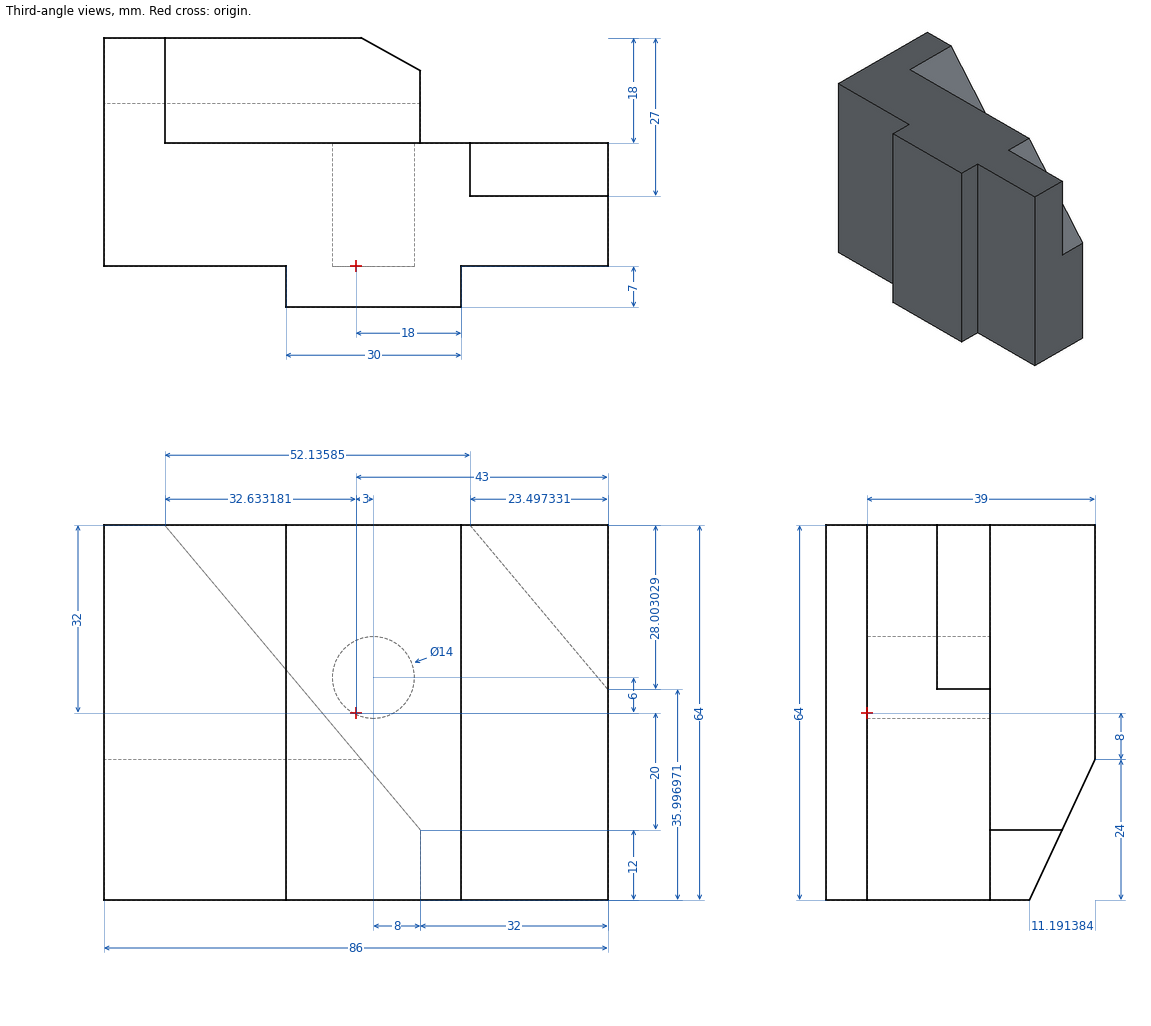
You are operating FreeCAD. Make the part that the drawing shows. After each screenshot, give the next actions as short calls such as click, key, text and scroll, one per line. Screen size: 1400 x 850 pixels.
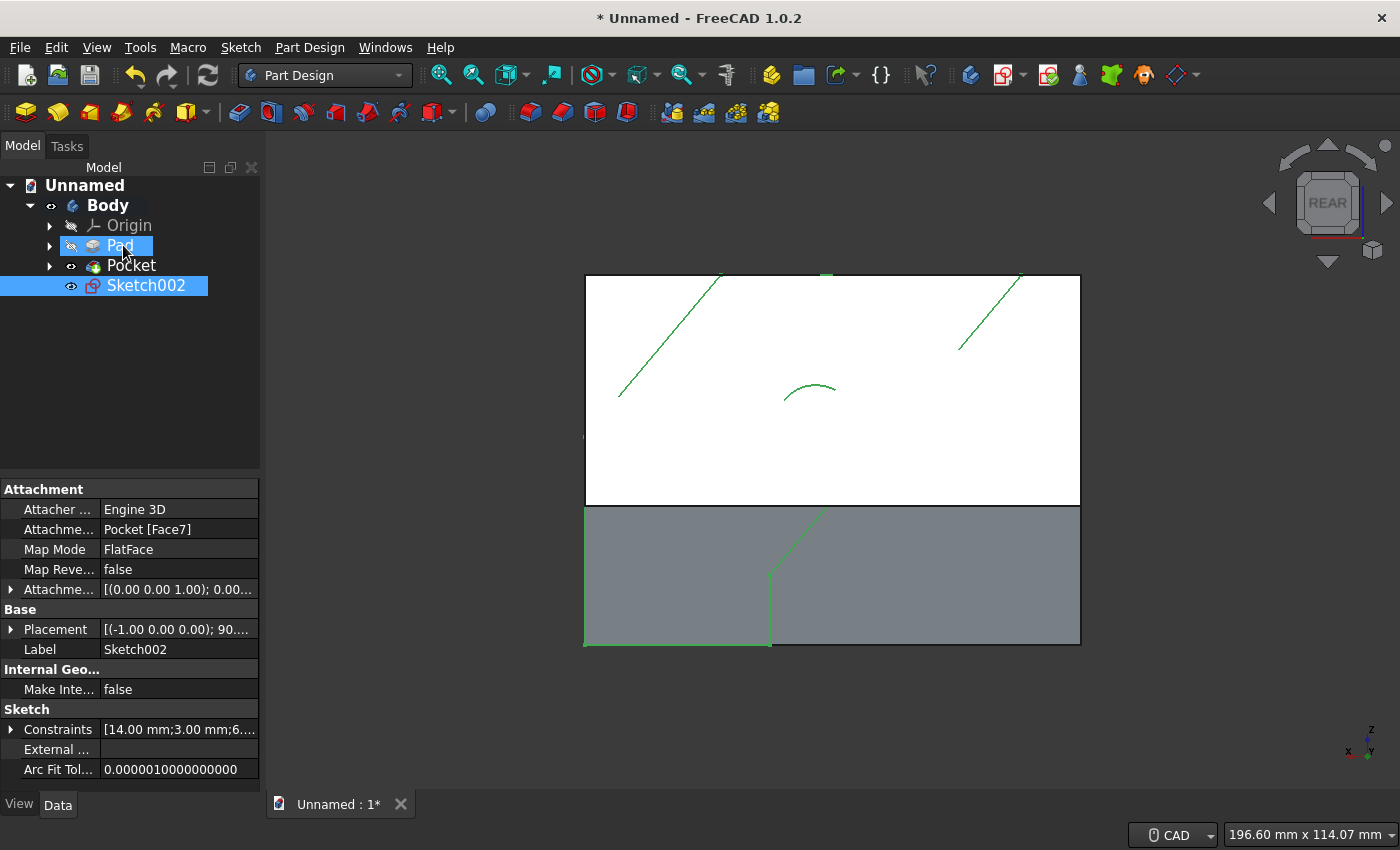
click(240, 112)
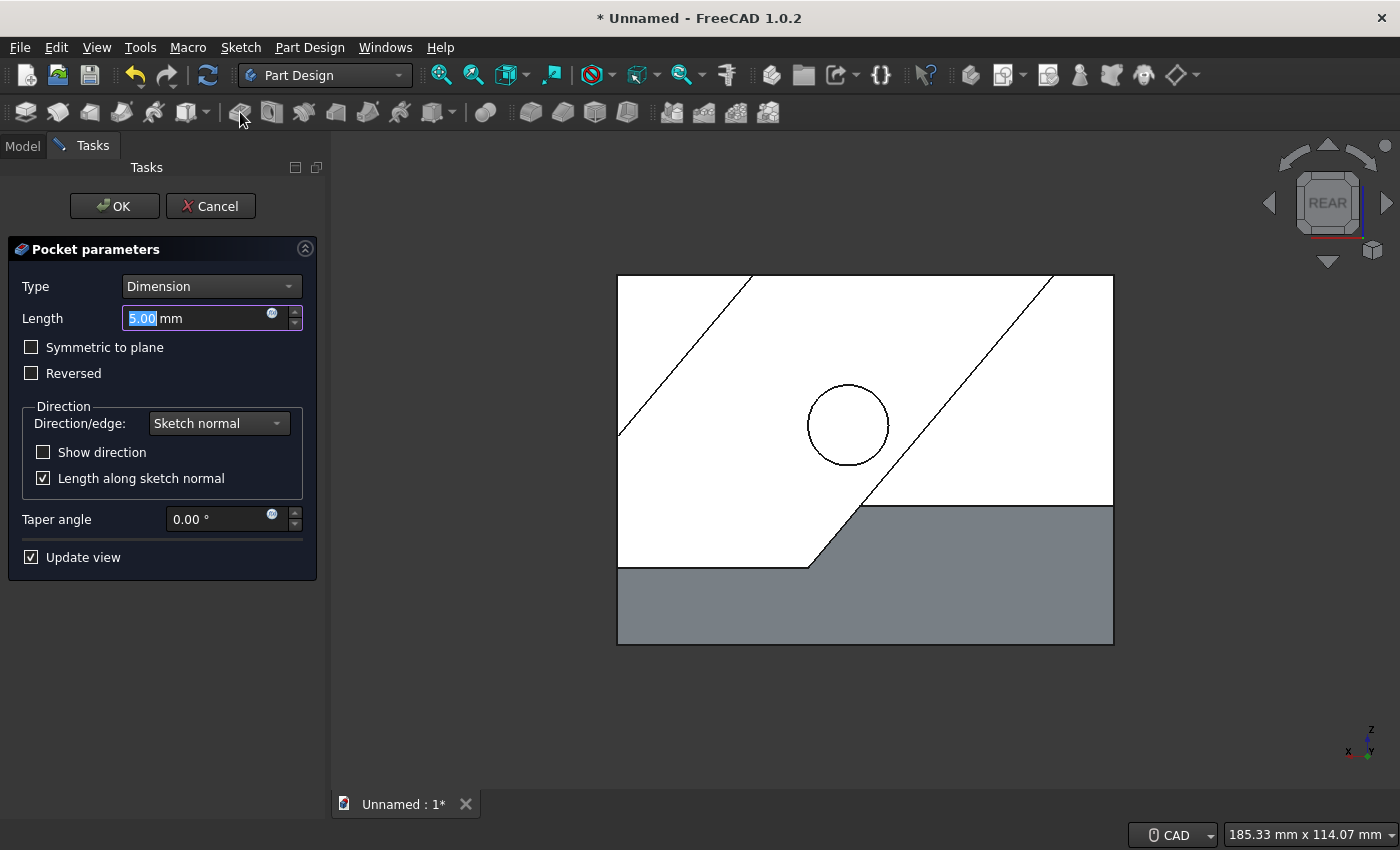
text(18)
key(Tab)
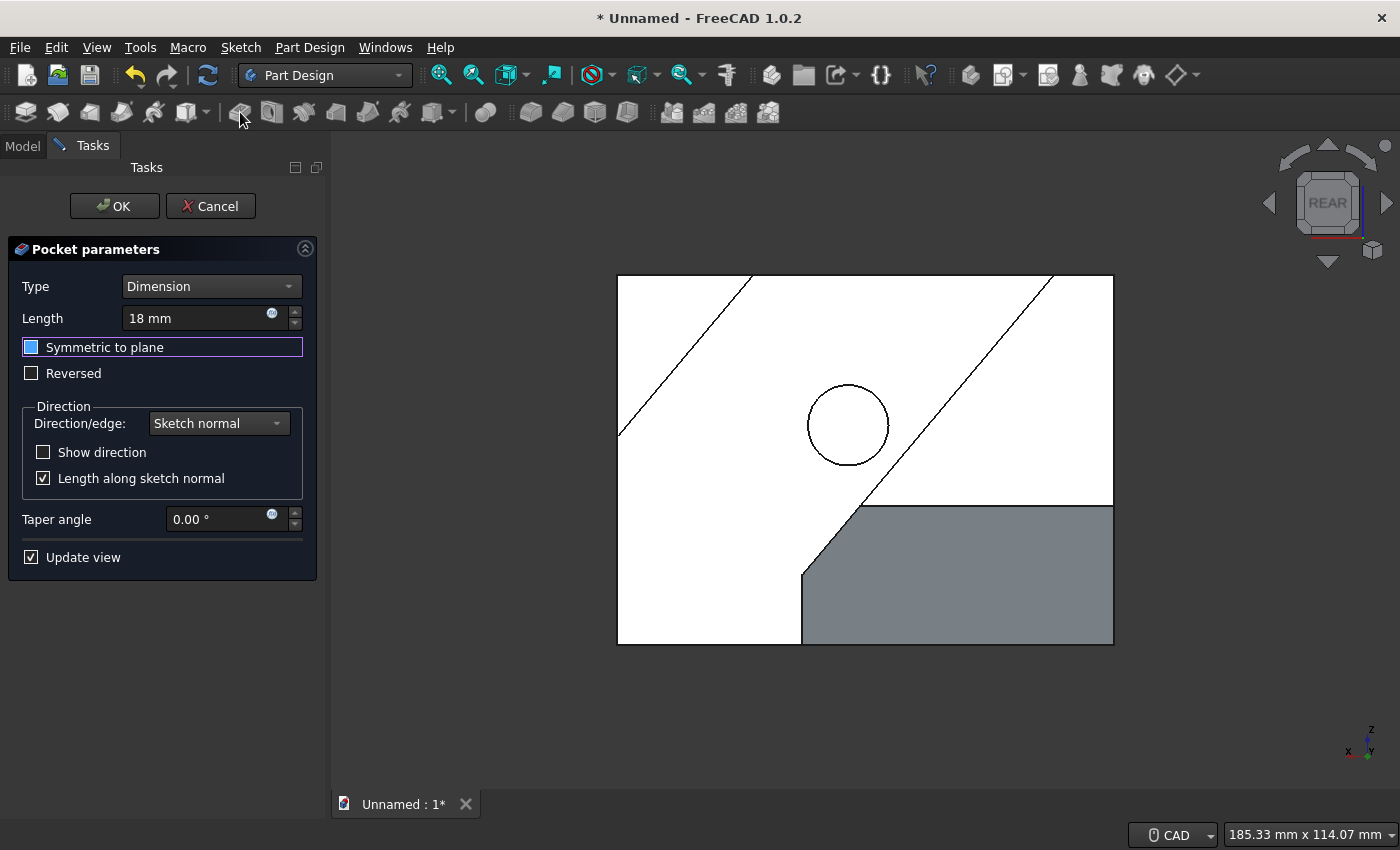
click(115, 206)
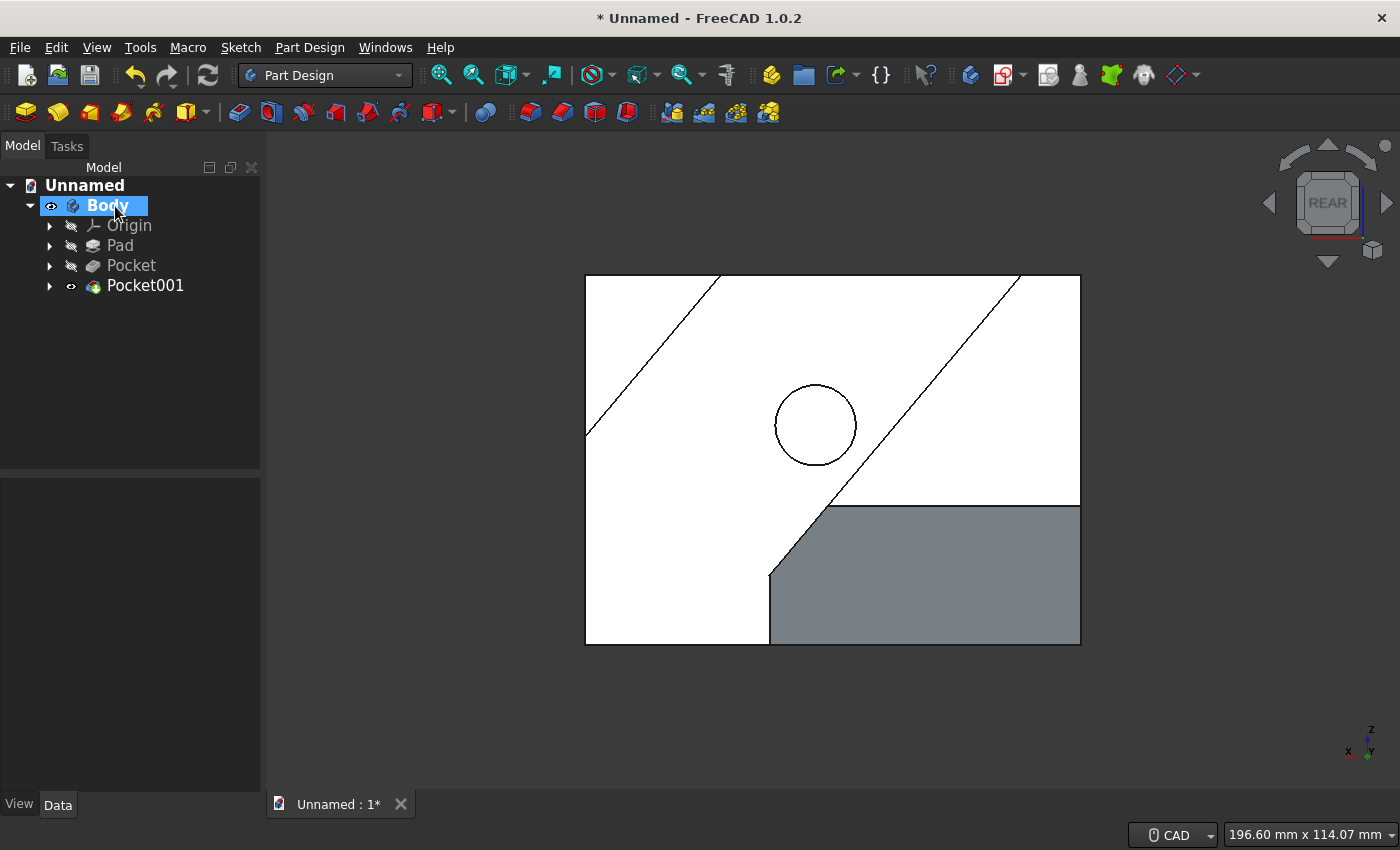
click(991, 423)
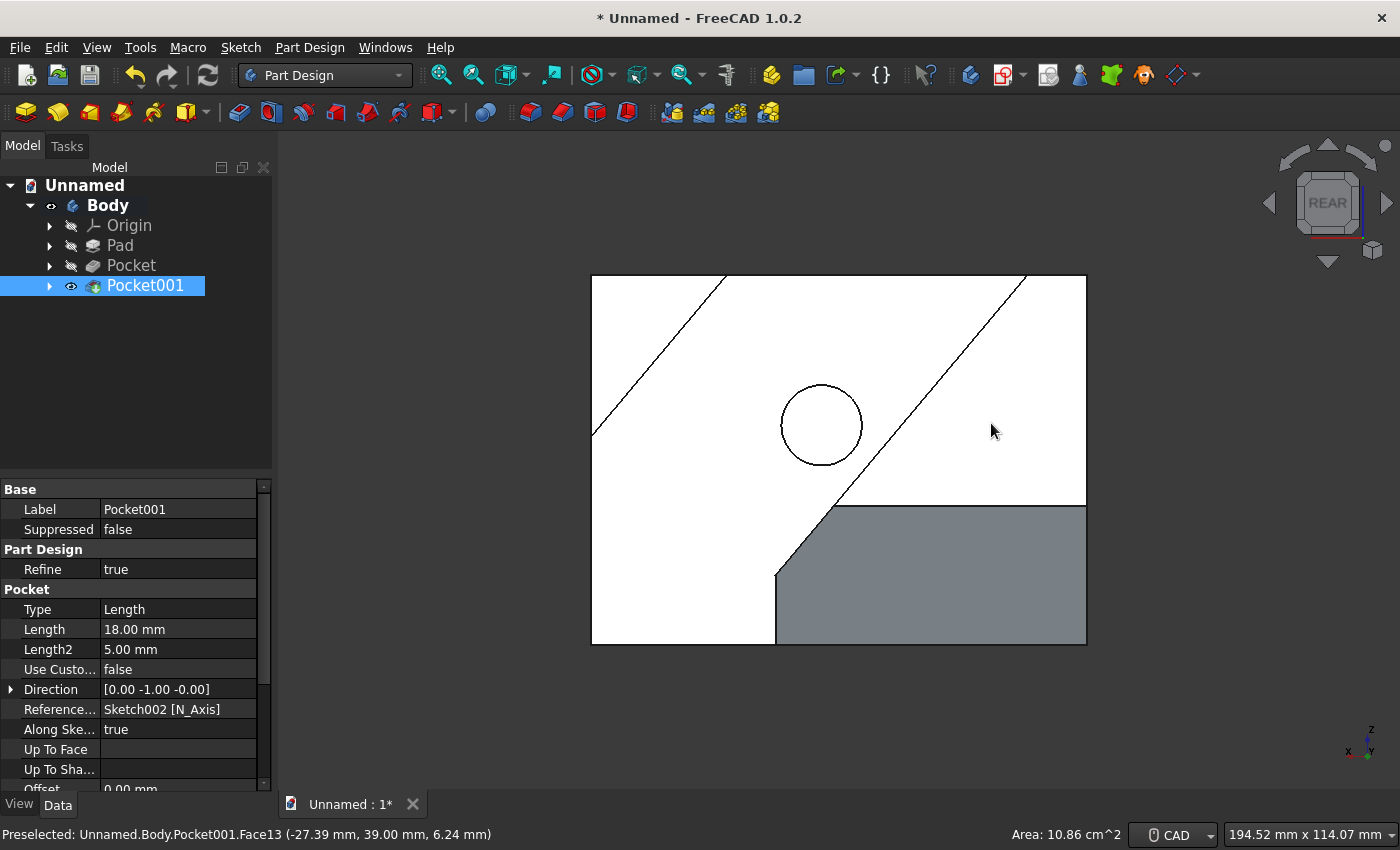
click(1004, 76)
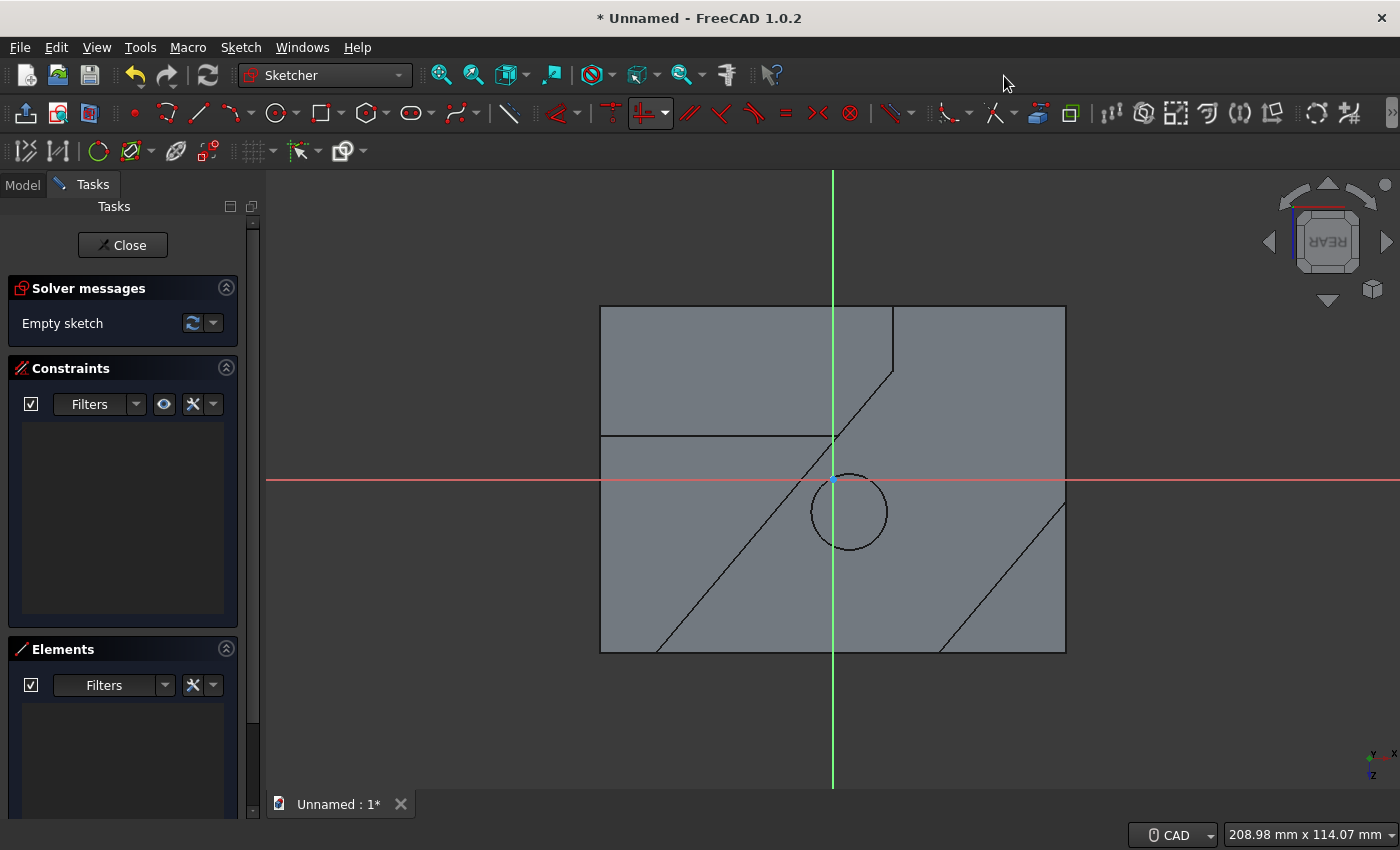
scroll(1101, 637, up, 4)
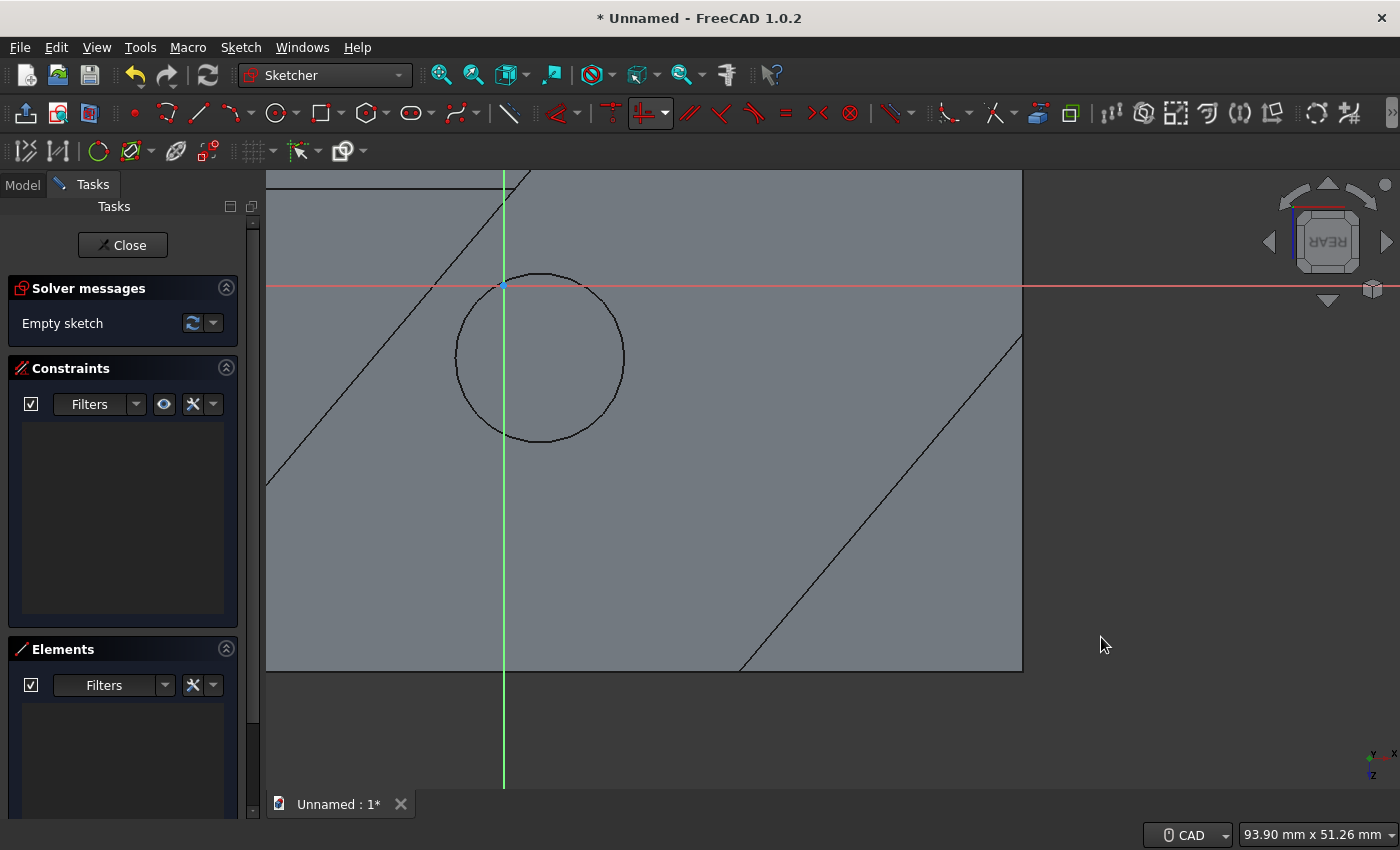
key(g)
key(m)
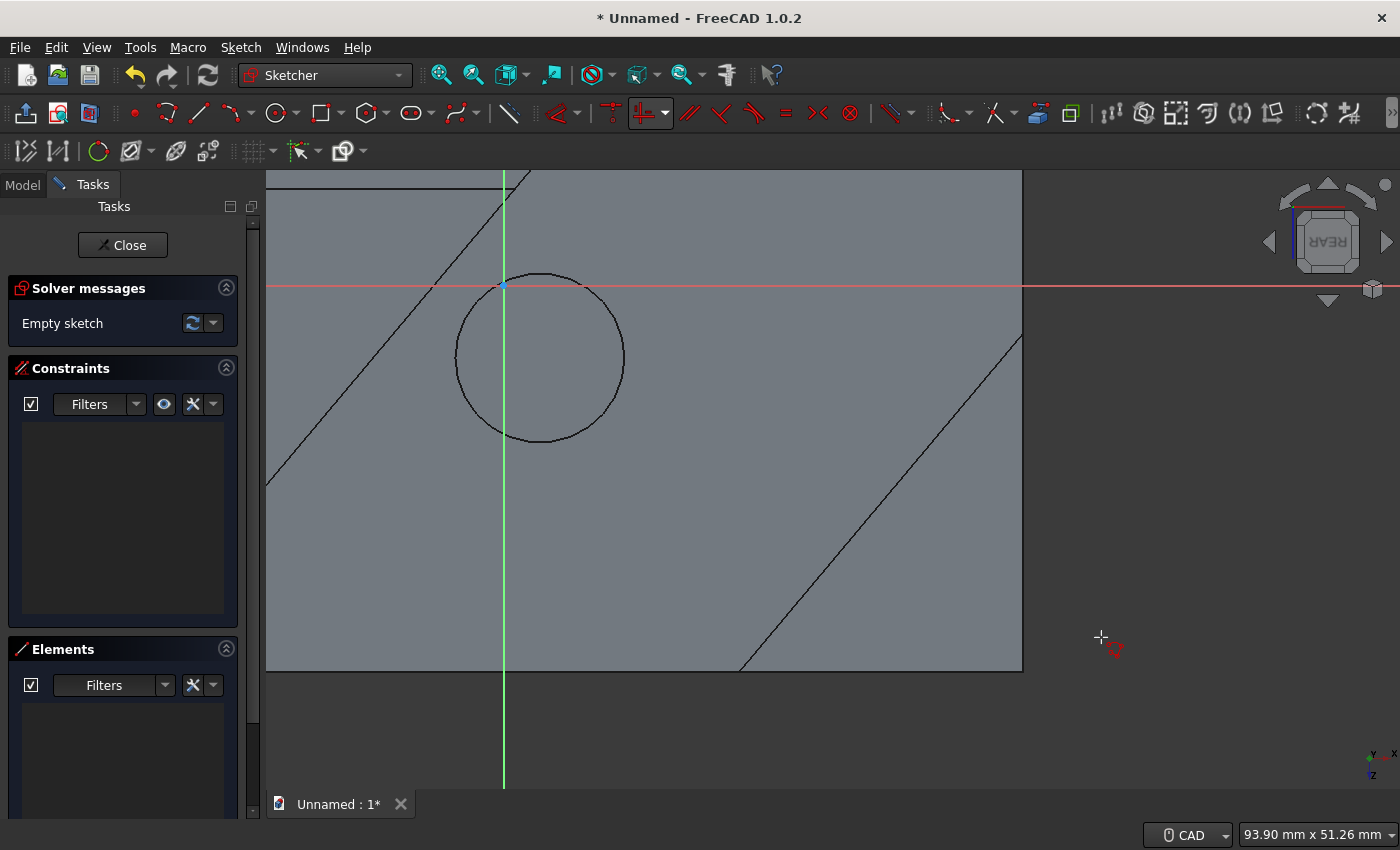
click(739, 672)
click(1023, 672)
click(1023, 334)
click(739, 673)
key(Escape)
key(Escape)